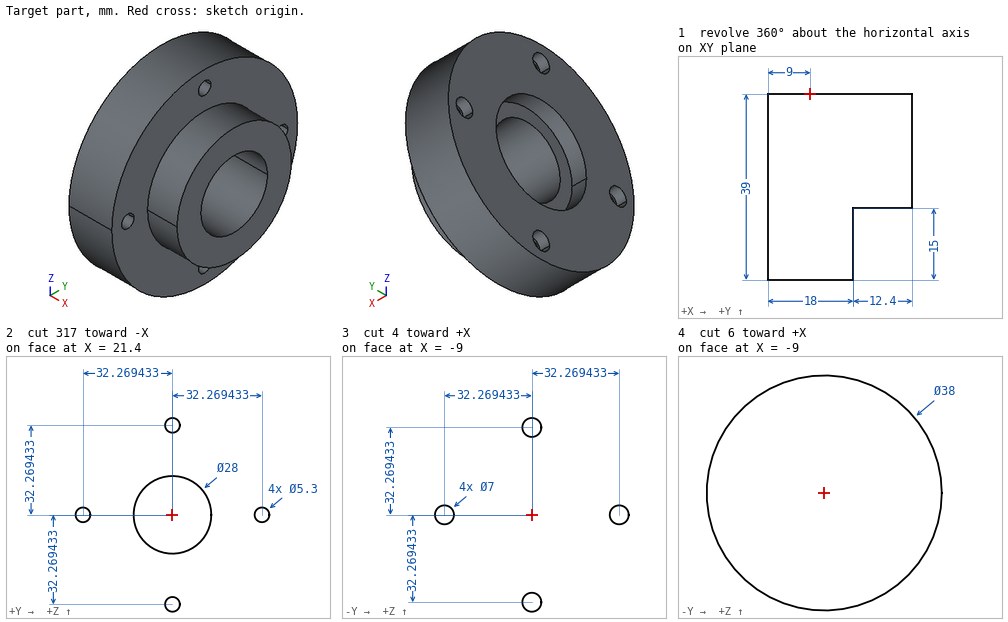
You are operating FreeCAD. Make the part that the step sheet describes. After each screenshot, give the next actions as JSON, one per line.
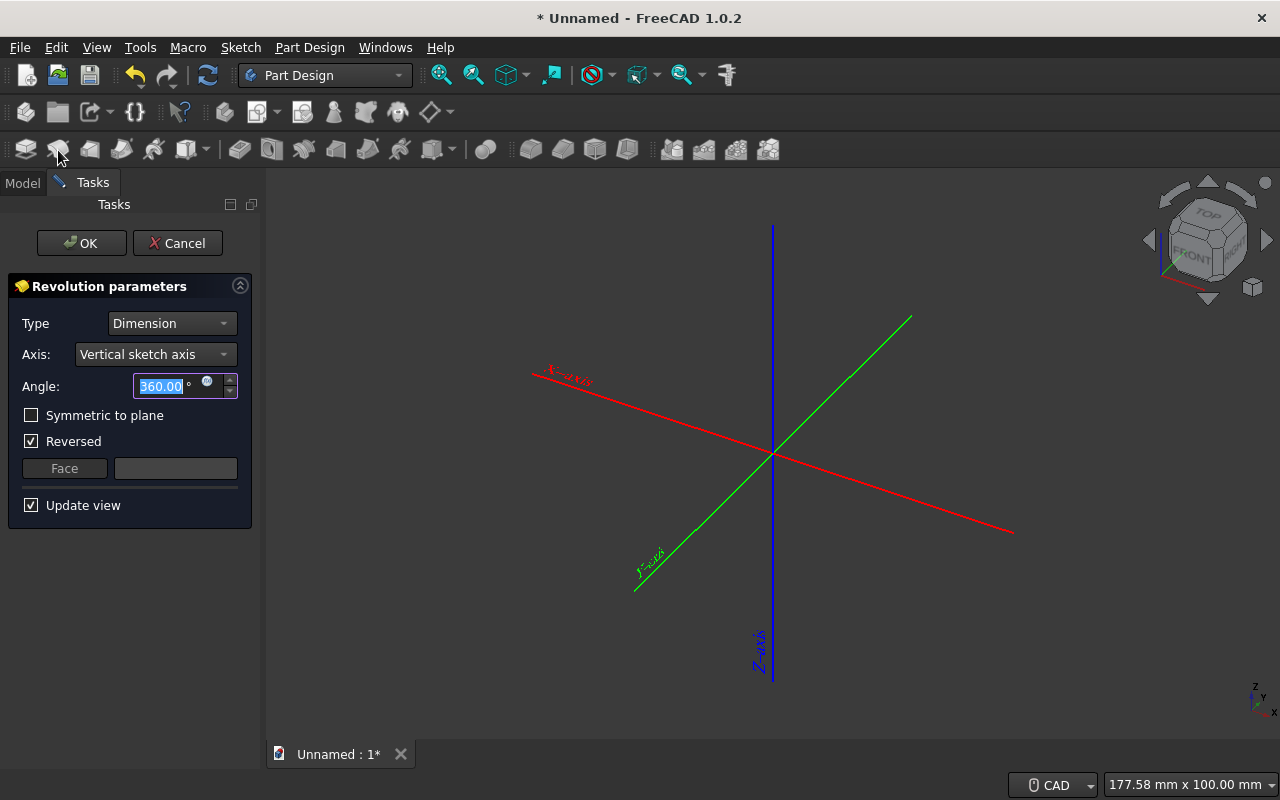
{"action": "left_click", "coordinate": [156, 354]}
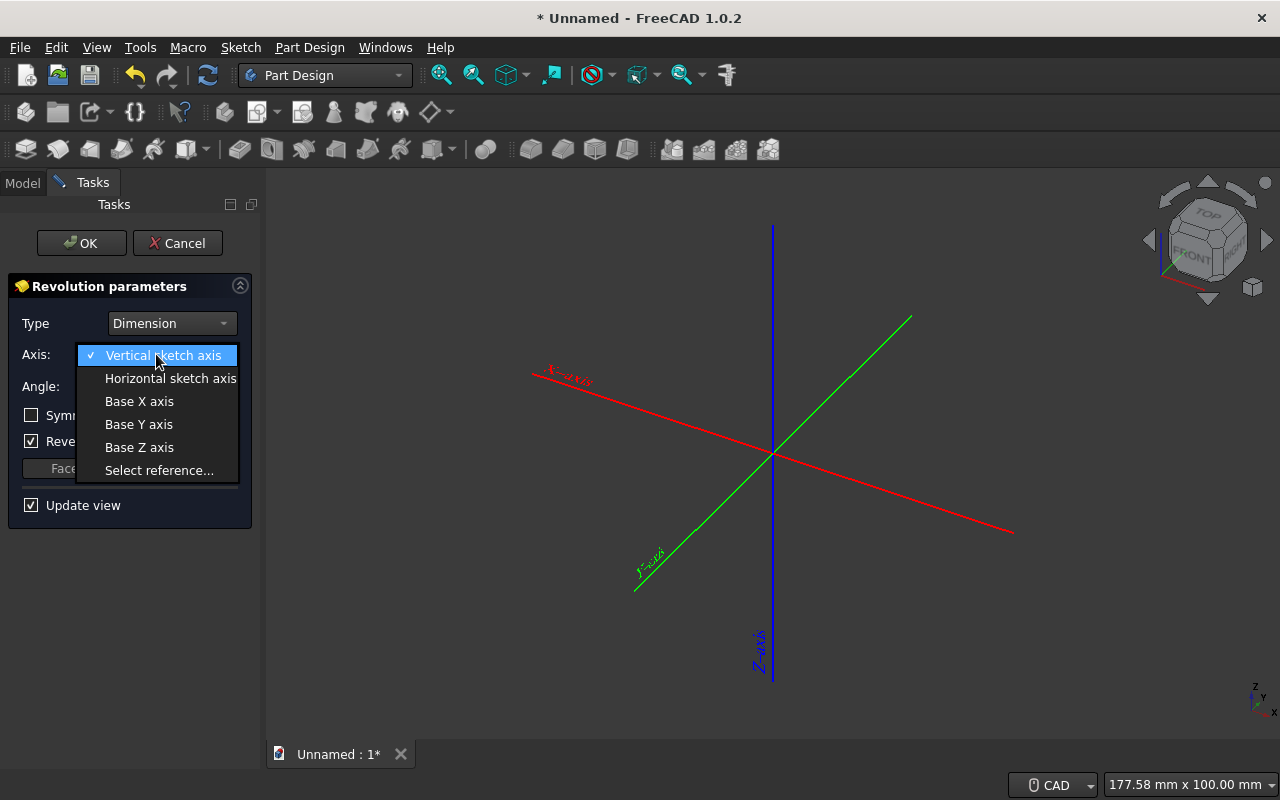
{"action": "left_click", "coordinate": [156, 378]}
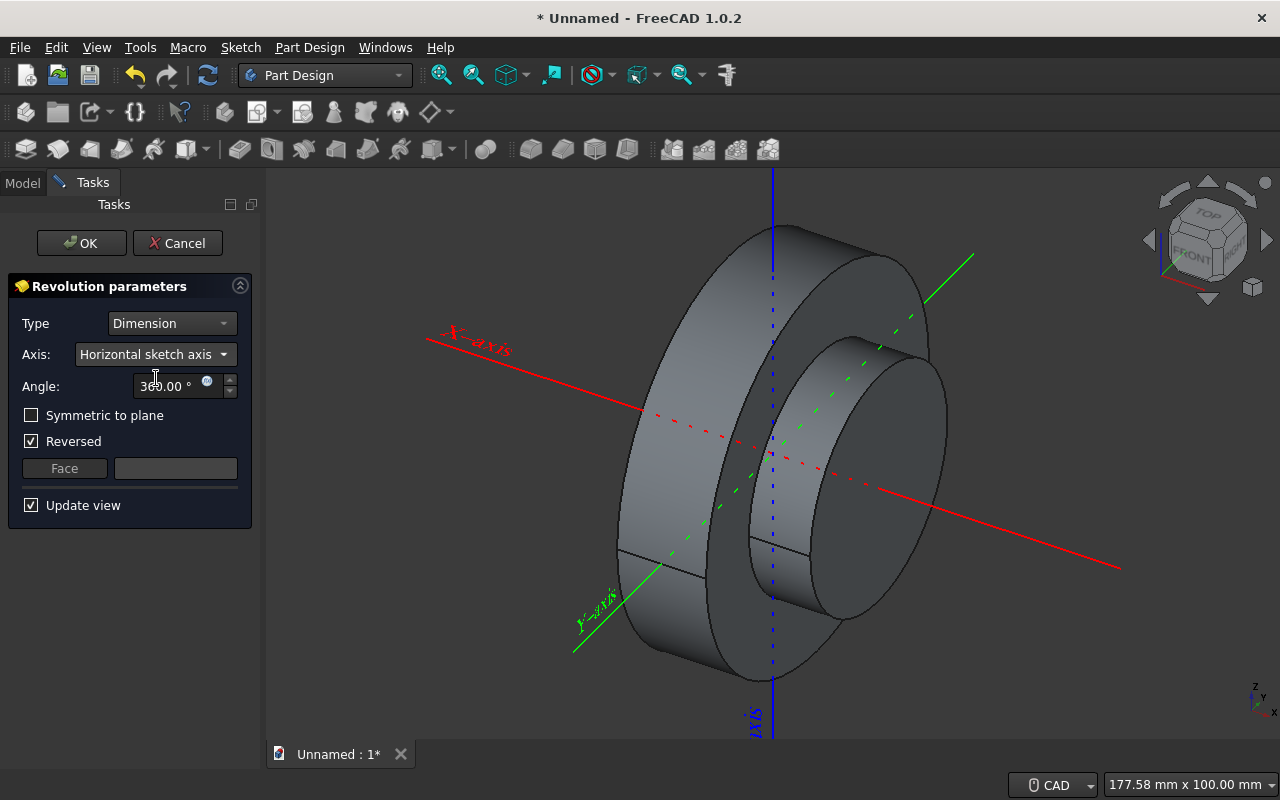
{"action": "left_click", "coordinate": [82, 243]}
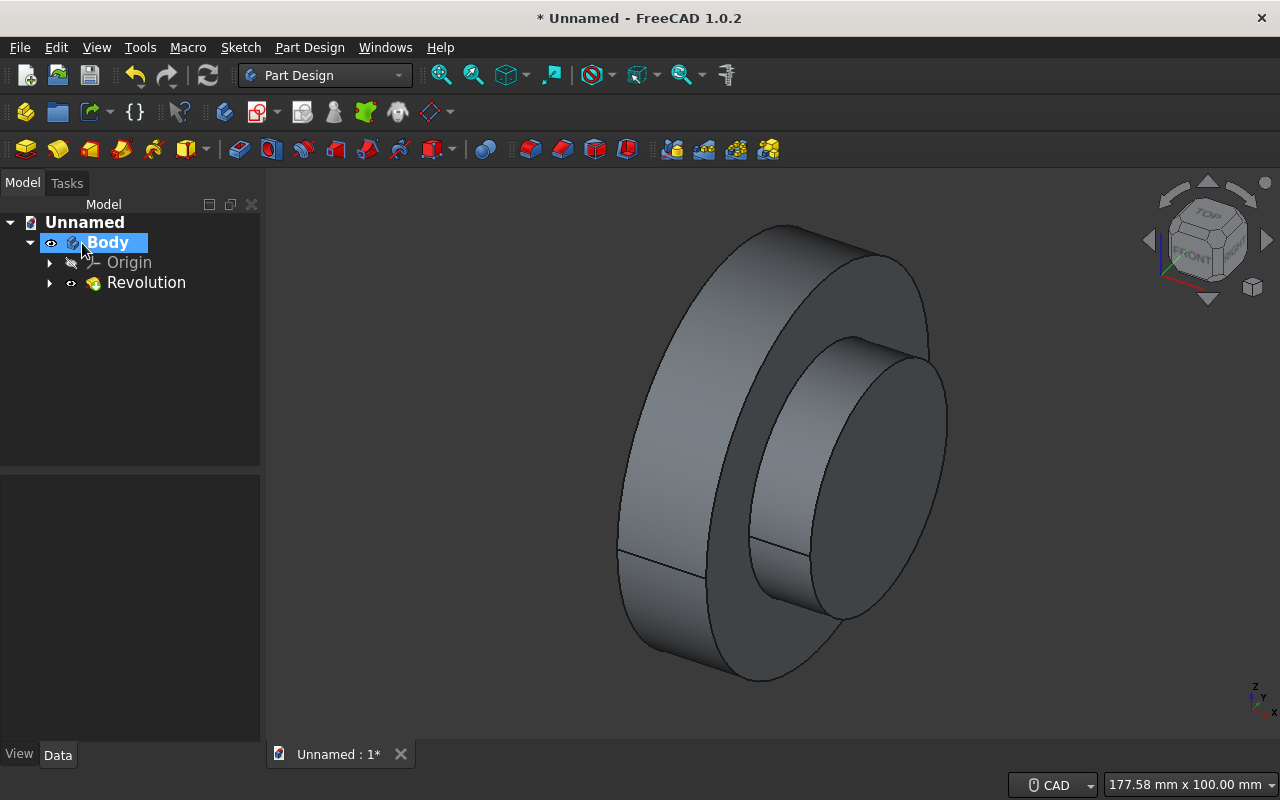
{"action": "left_click", "coordinate": [442, 76]}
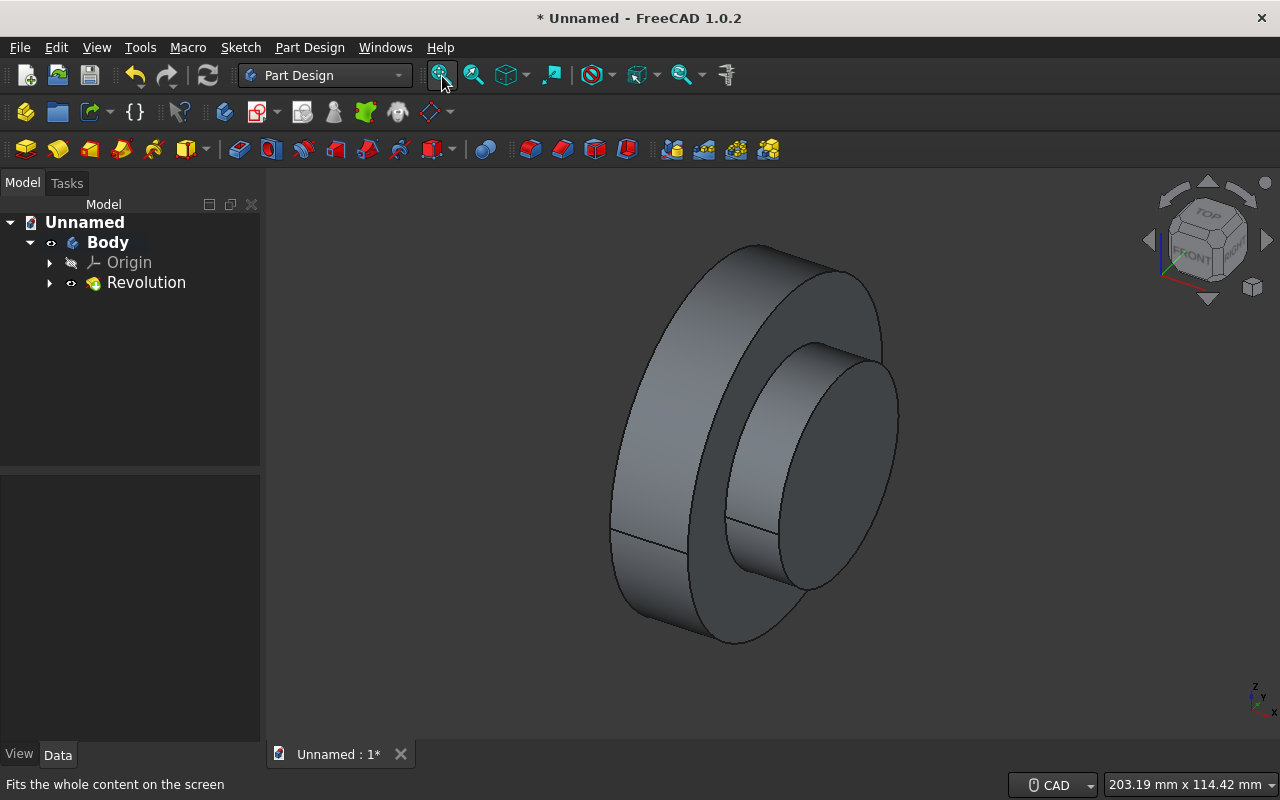
{"action": "left_click", "coordinate": [839, 474]}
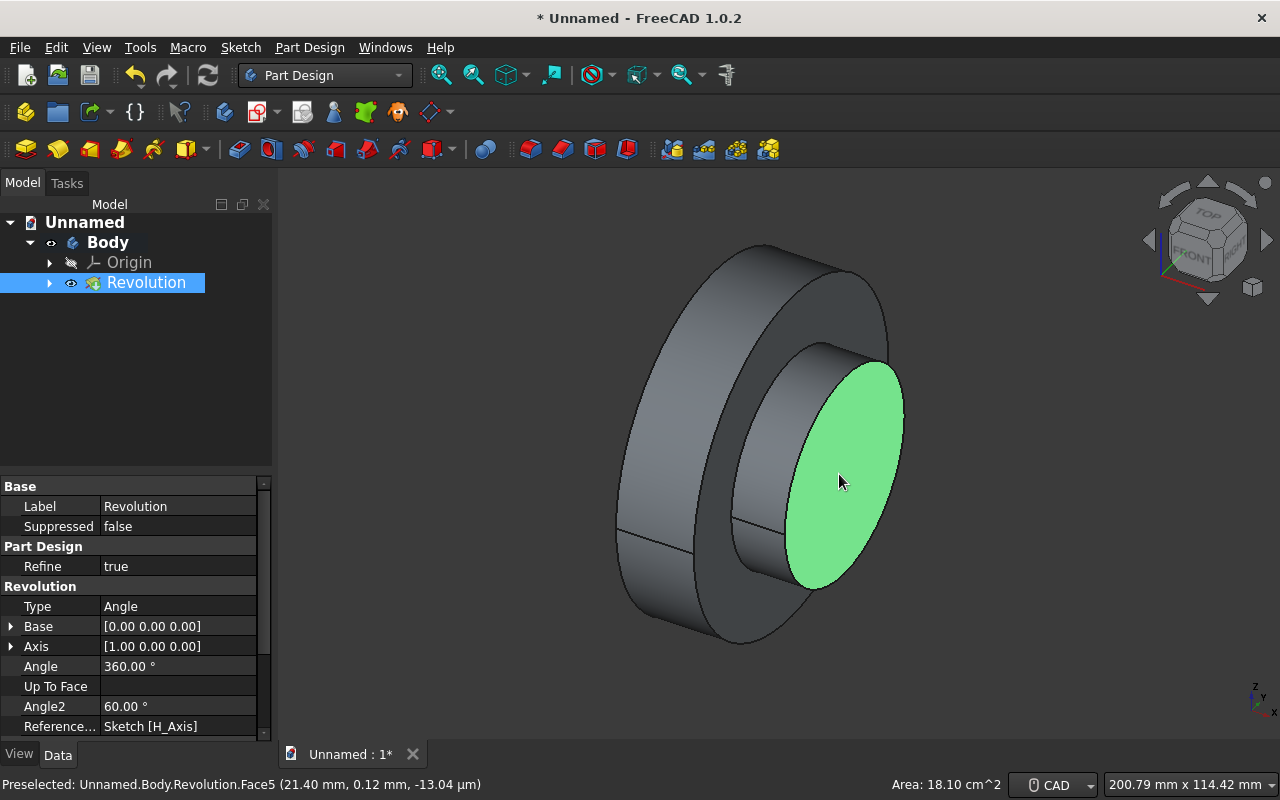
{"action": "left_click", "coordinate": [258, 112]}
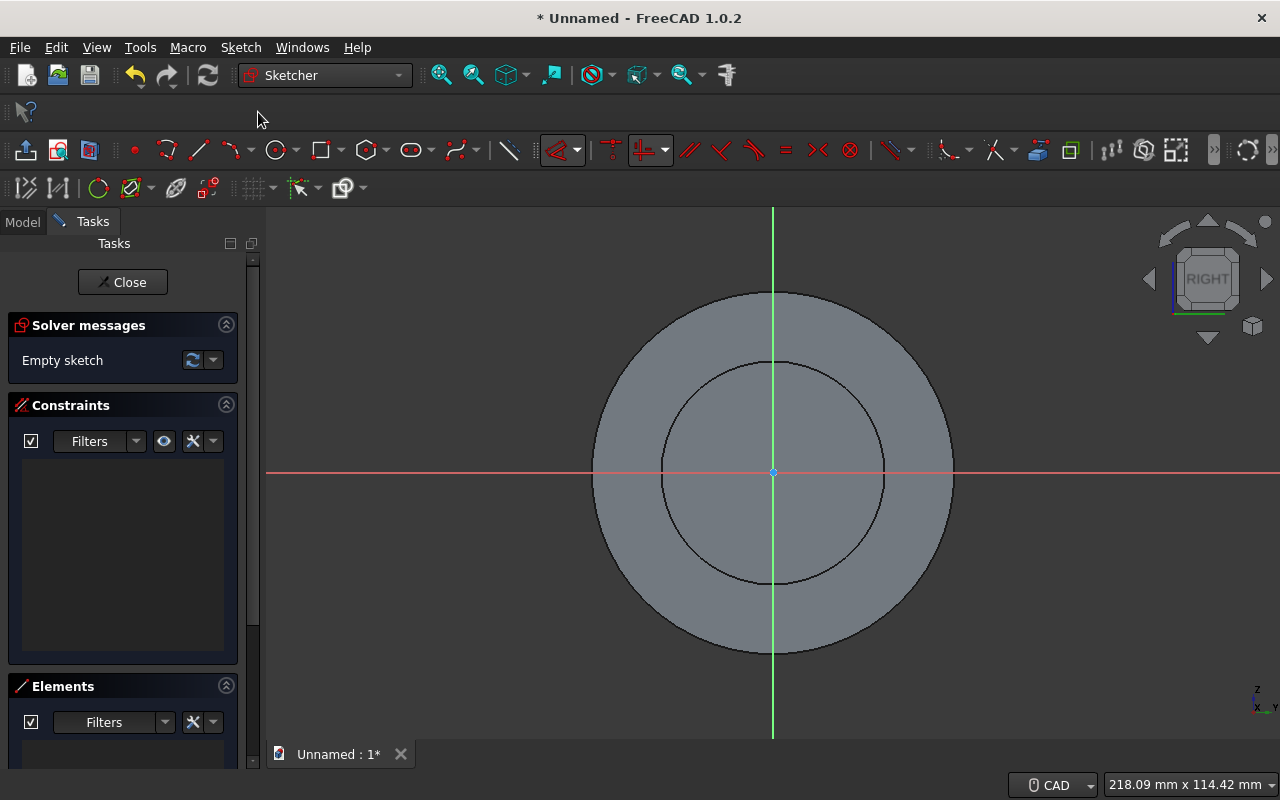
{"action": "key", "text": "g c"}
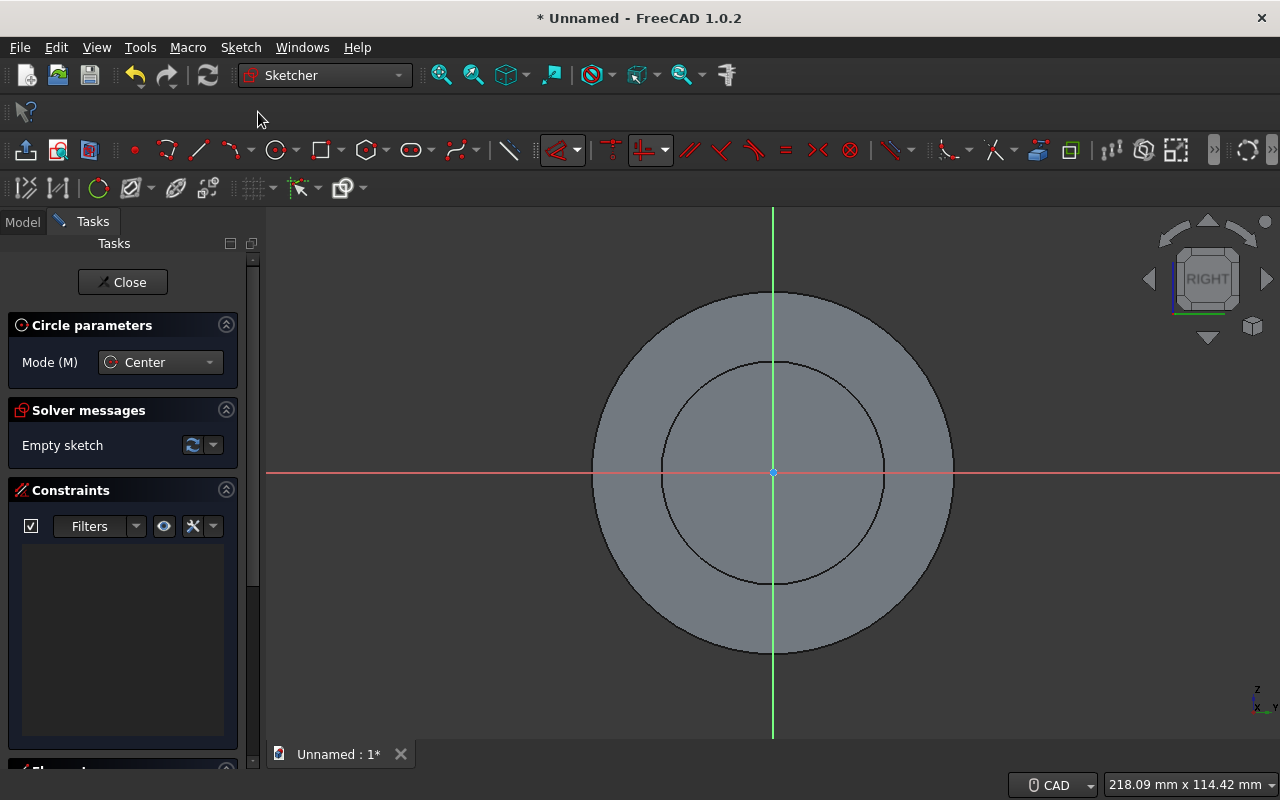
{"action": "left_click", "coordinate": [773, 473]}
{"action": "left_click", "coordinate": [819, 427]}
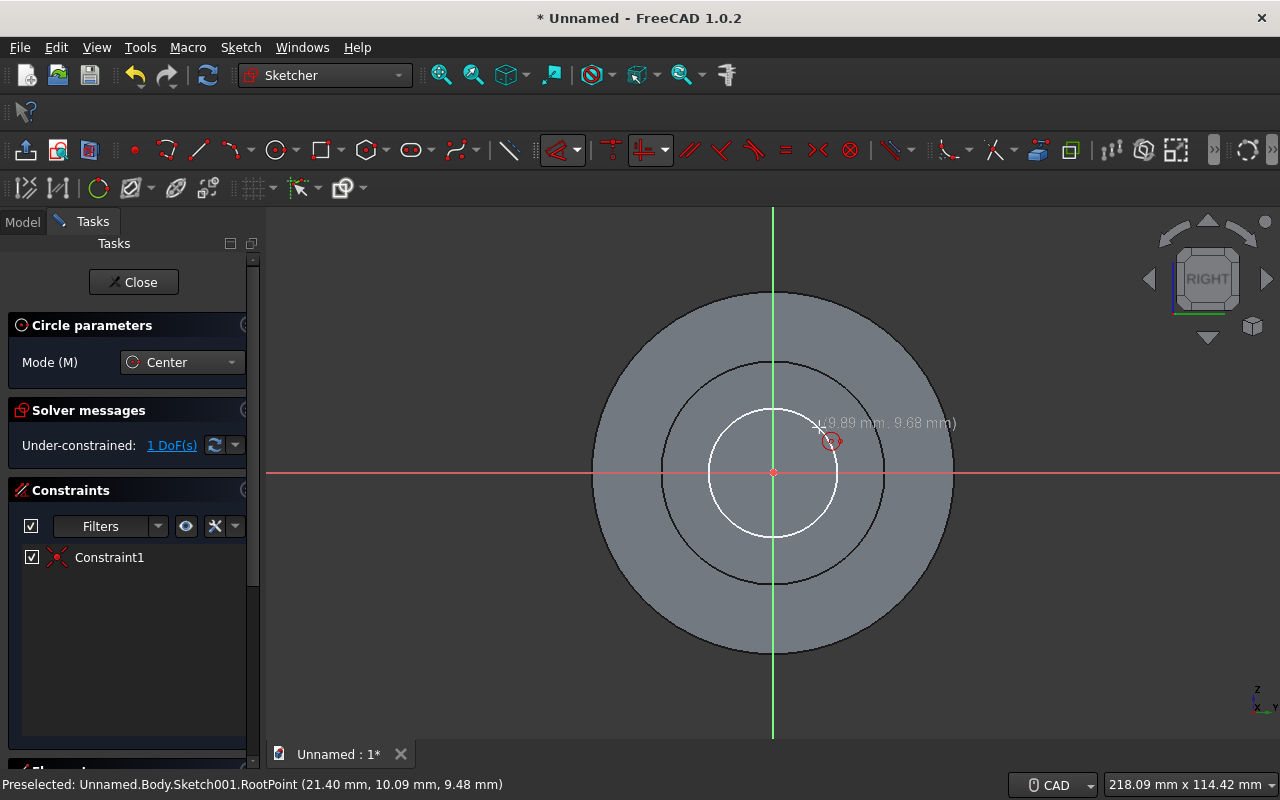
{"action": "scroll", "coordinate": [923, 473], "scroll_direction": "up", "scroll_amount": 4}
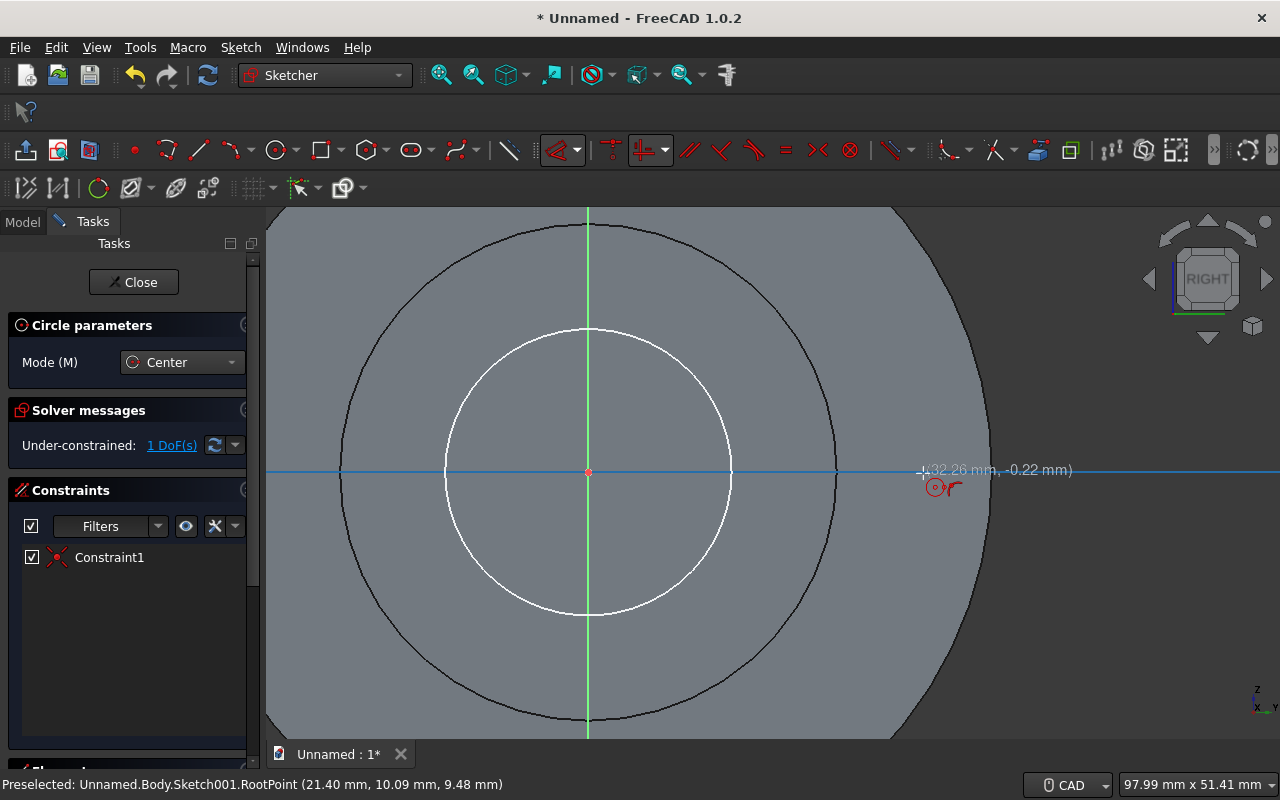
{"action": "left_click", "coordinate": [922, 472]}
{"action": "left_click", "coordinate": [942, 453]}